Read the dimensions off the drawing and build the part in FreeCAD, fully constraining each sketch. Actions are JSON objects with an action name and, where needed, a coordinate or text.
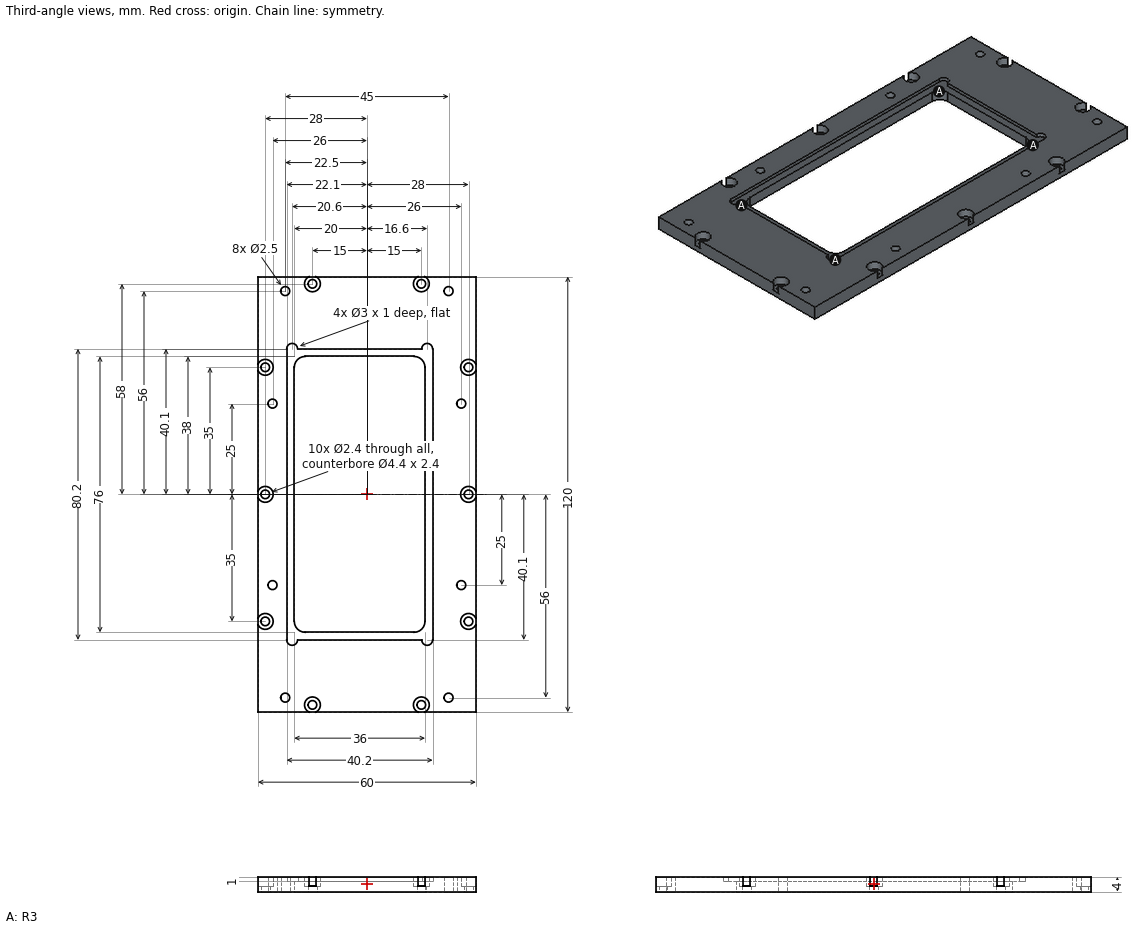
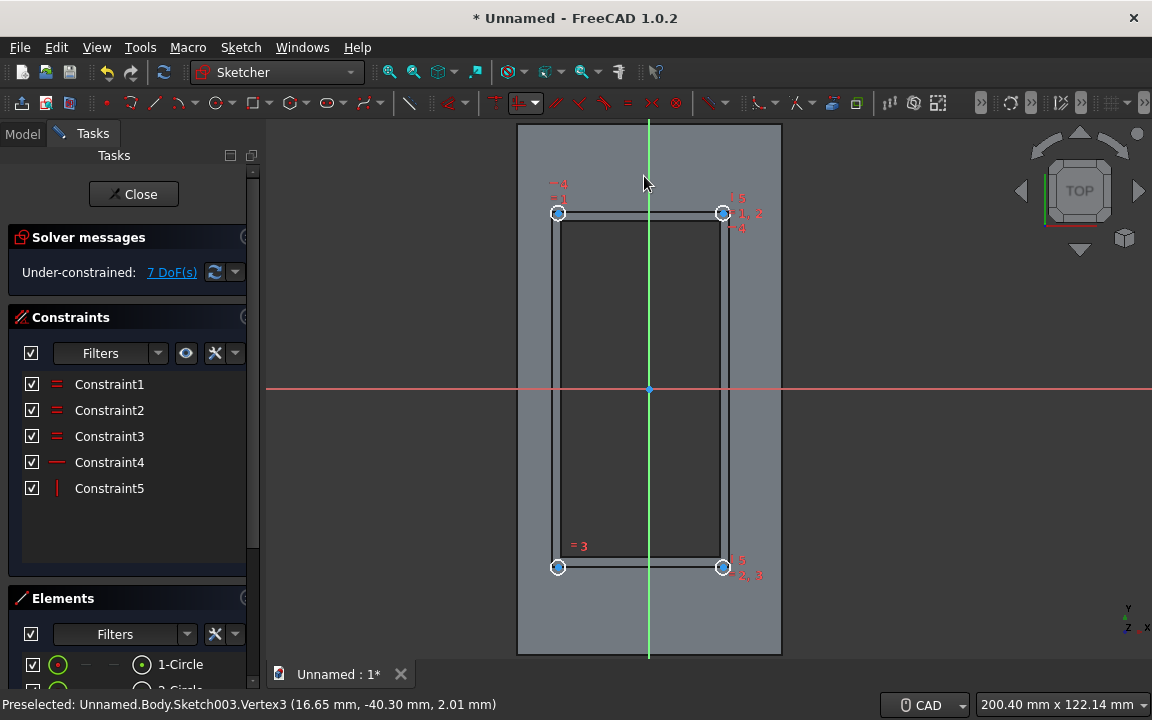
{"action": "left_click", "coordinate": [558, 213]}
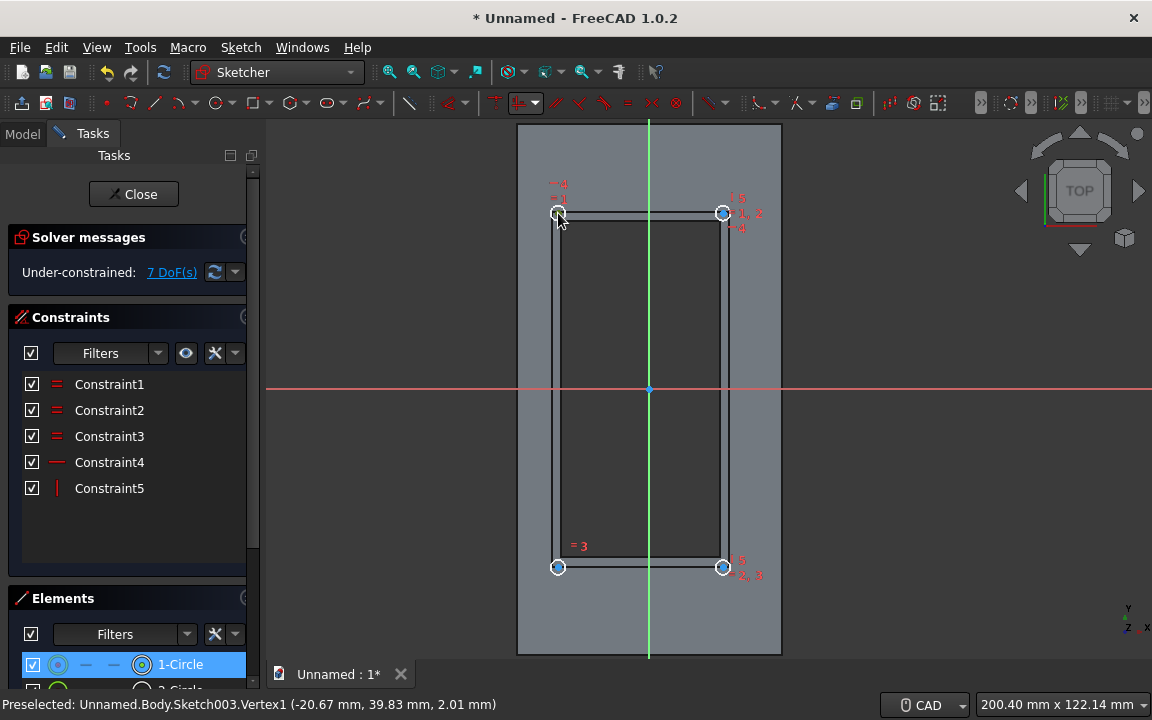
{"action": "left_click", "coordinate": [558, 567]}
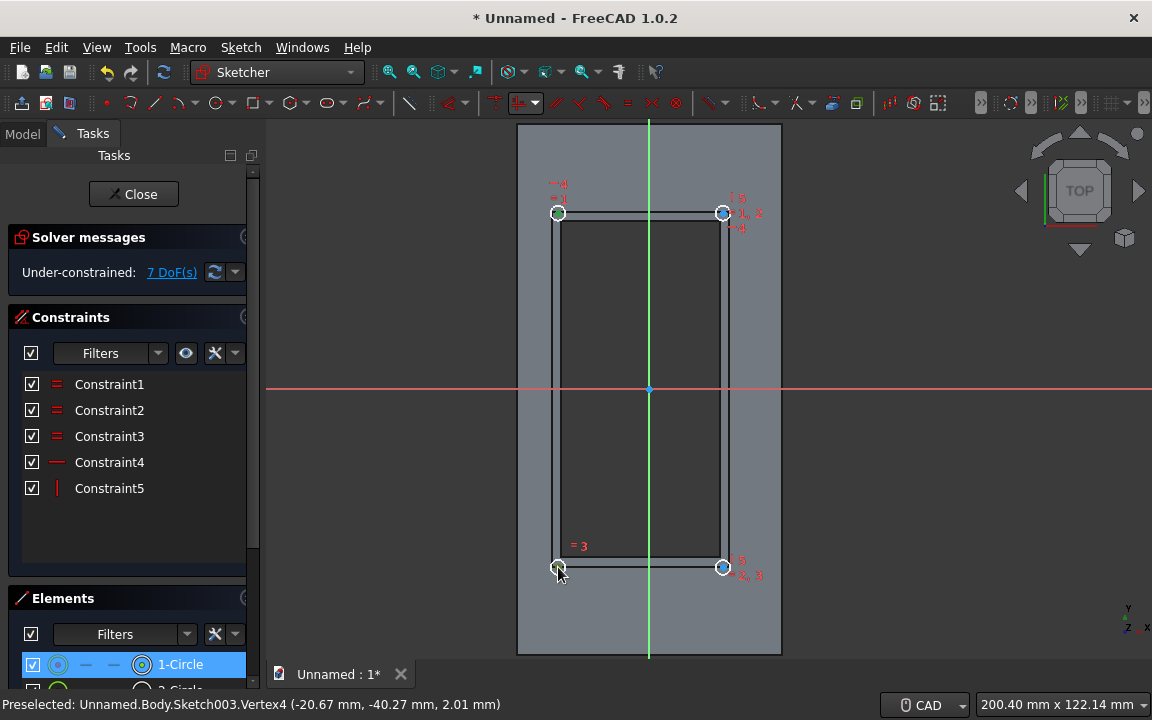
{"action": "key", "text": "v"}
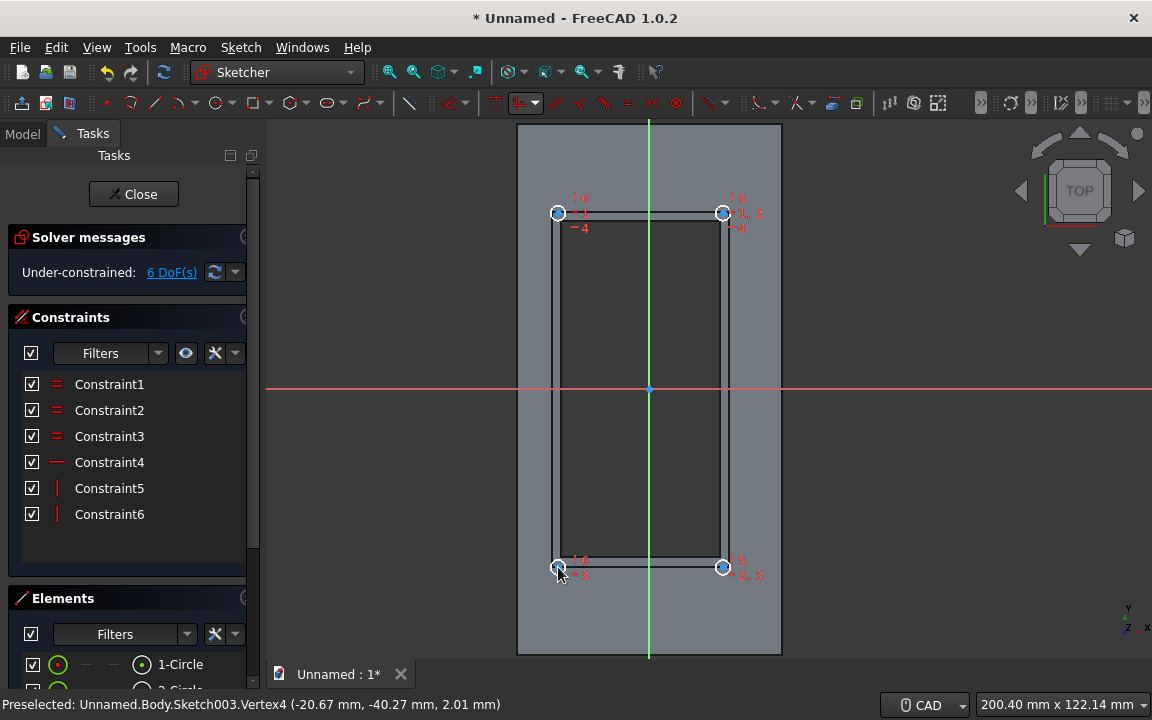
{"action": "left_click", "coordinate": [723, 567]}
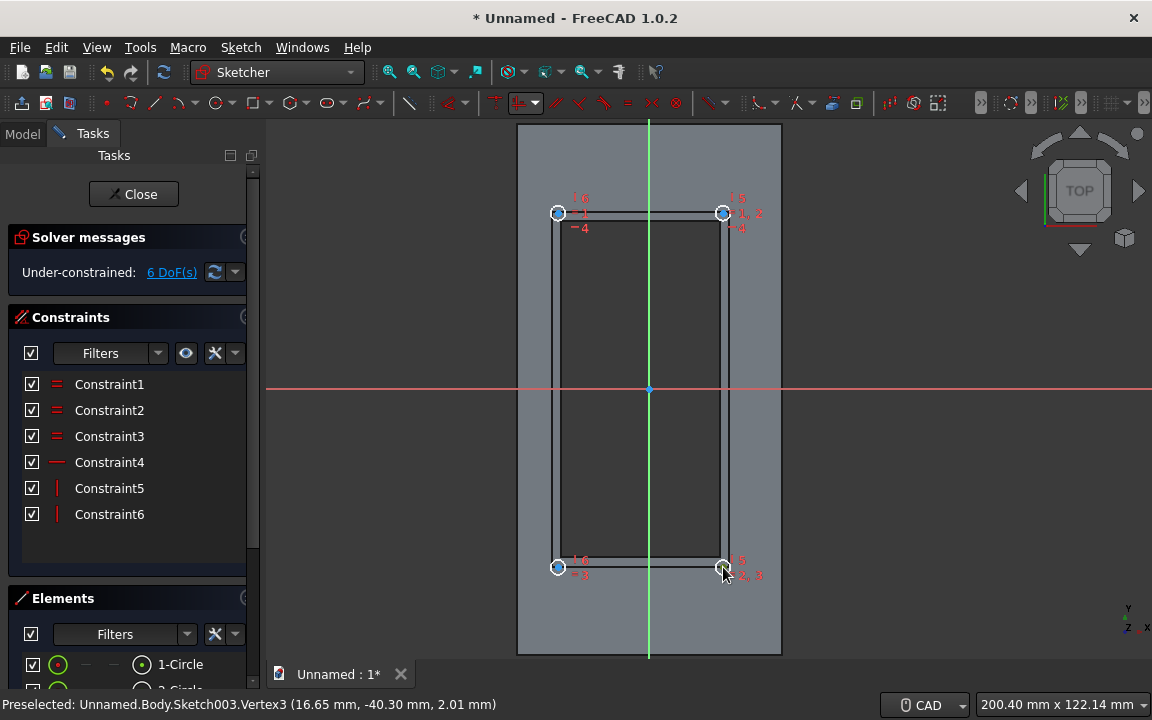
{"action": "left_click", "coordinate": [558, 567]}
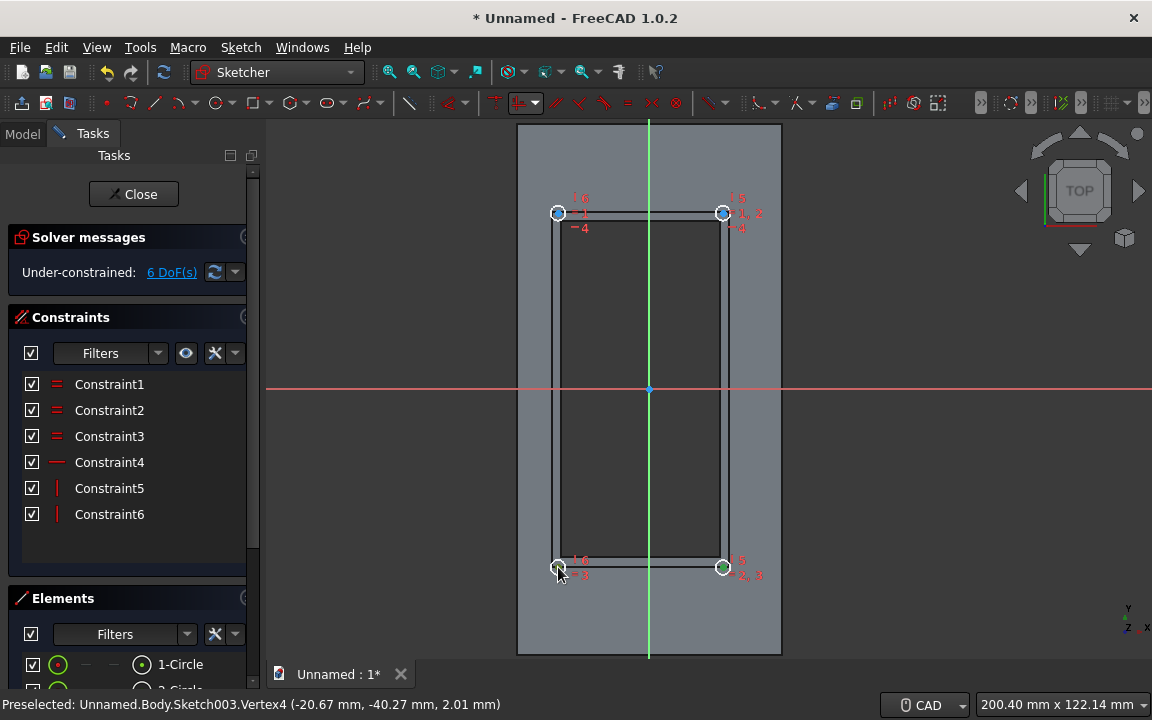
{"action": "key", "text": "h"}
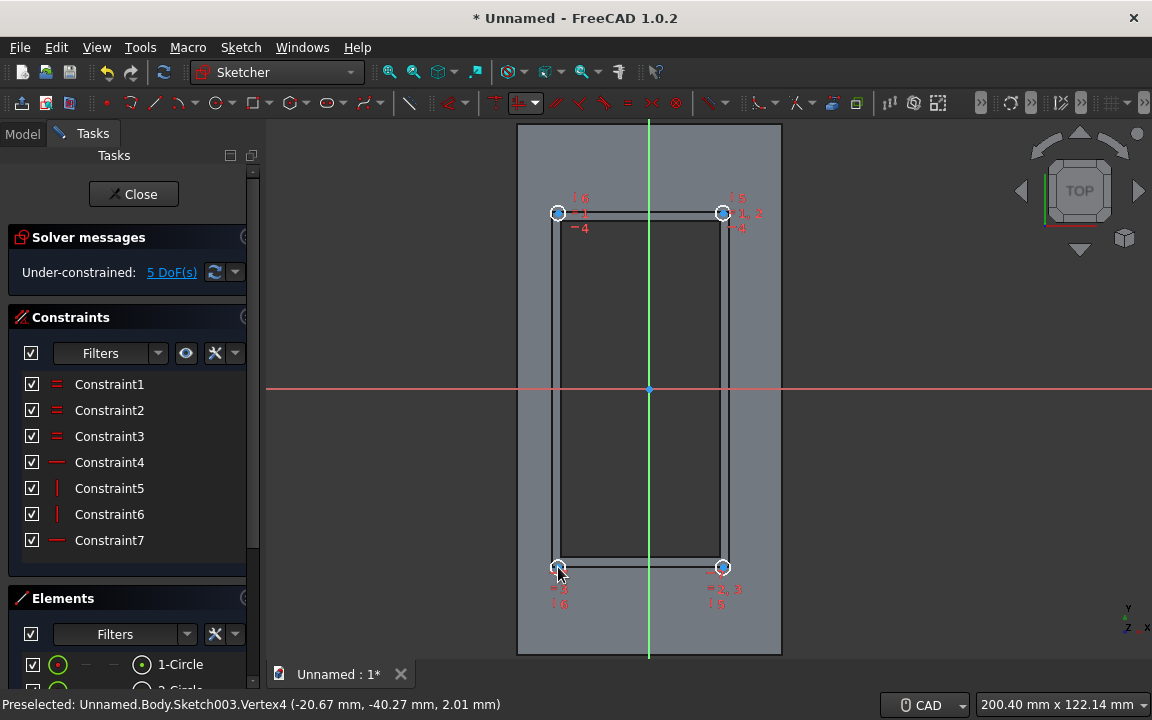
{"action": "key", "text": "d"}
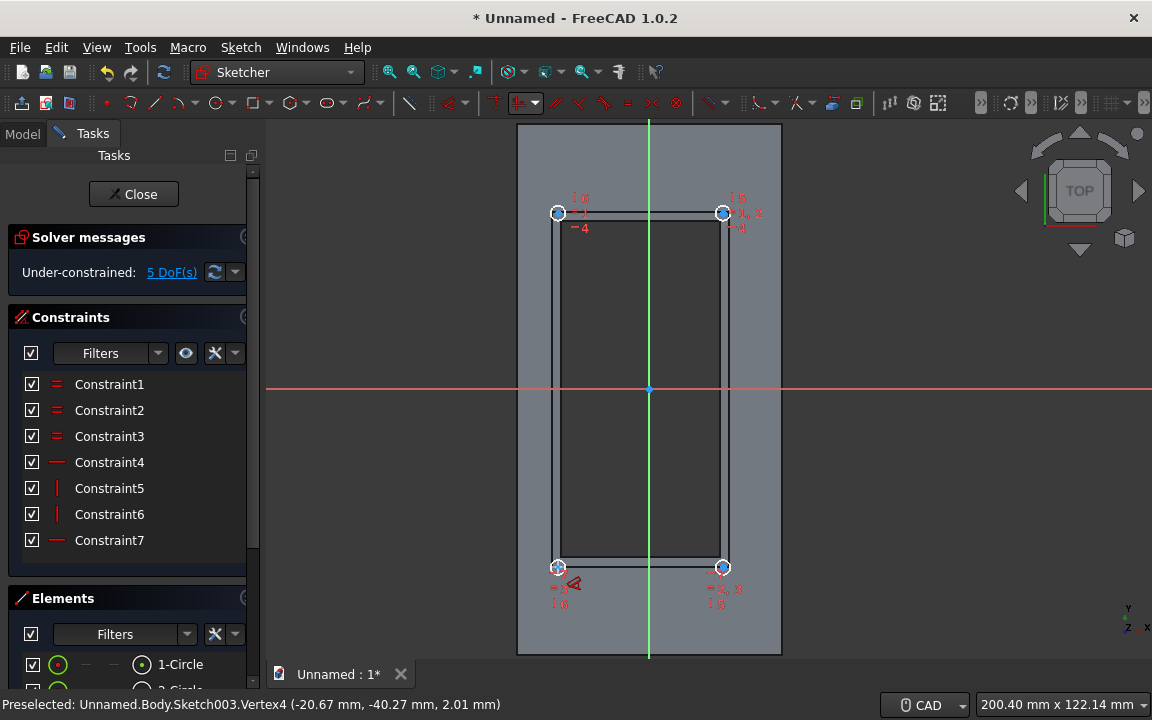
{"action": "scroll", "coordinate": [563, 218], "scroll_direction": "up", "scroll_amount": 6}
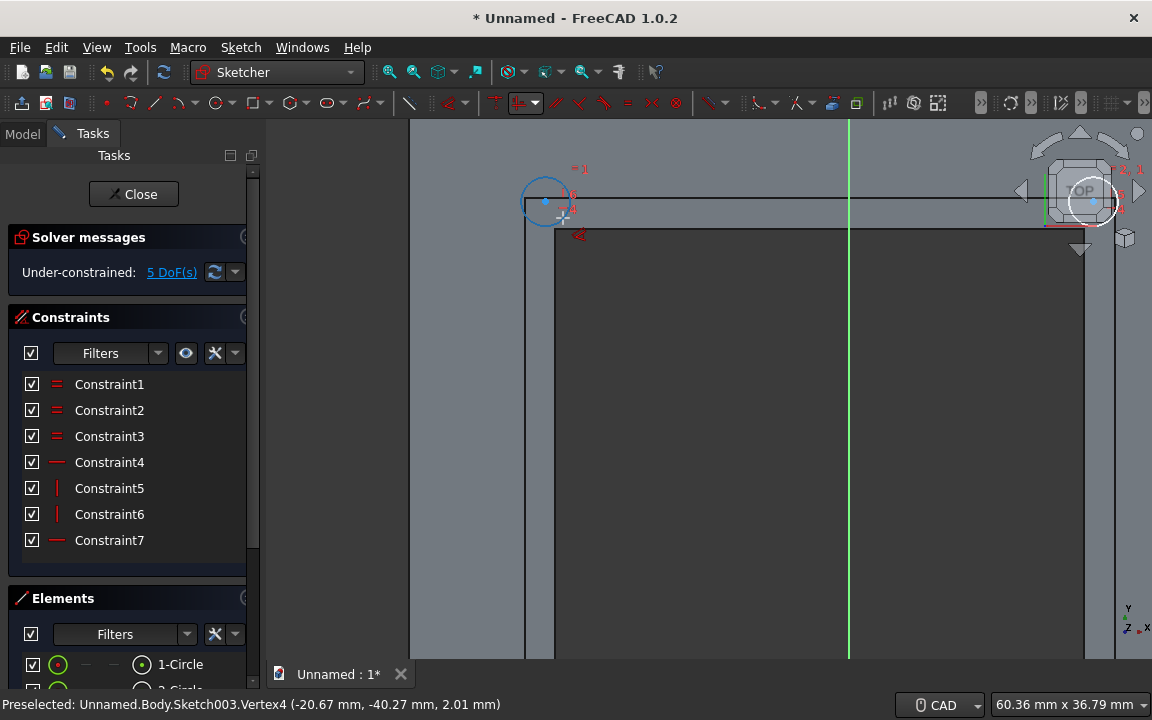
{"action": "left_click", "coordinate": [563, 219]}
{"action": "left_click", "coordinate": [586, 242]}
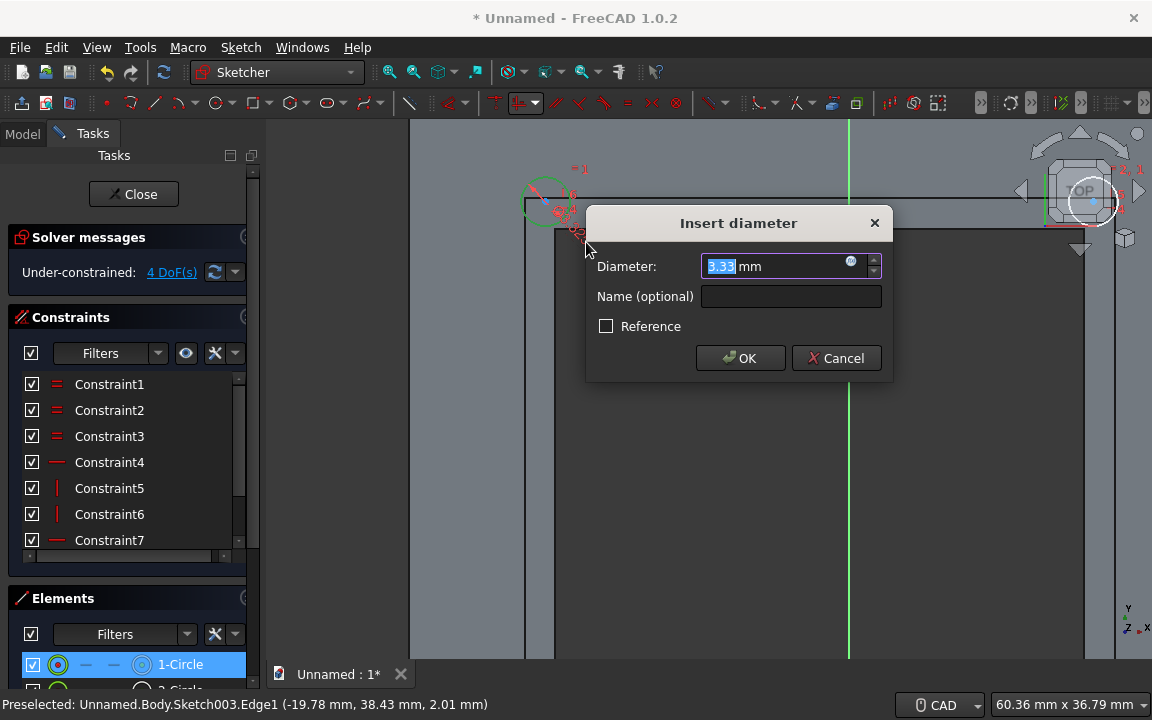
{"action": "type", "text": "3"}
{"action": "key", "text": "Return"}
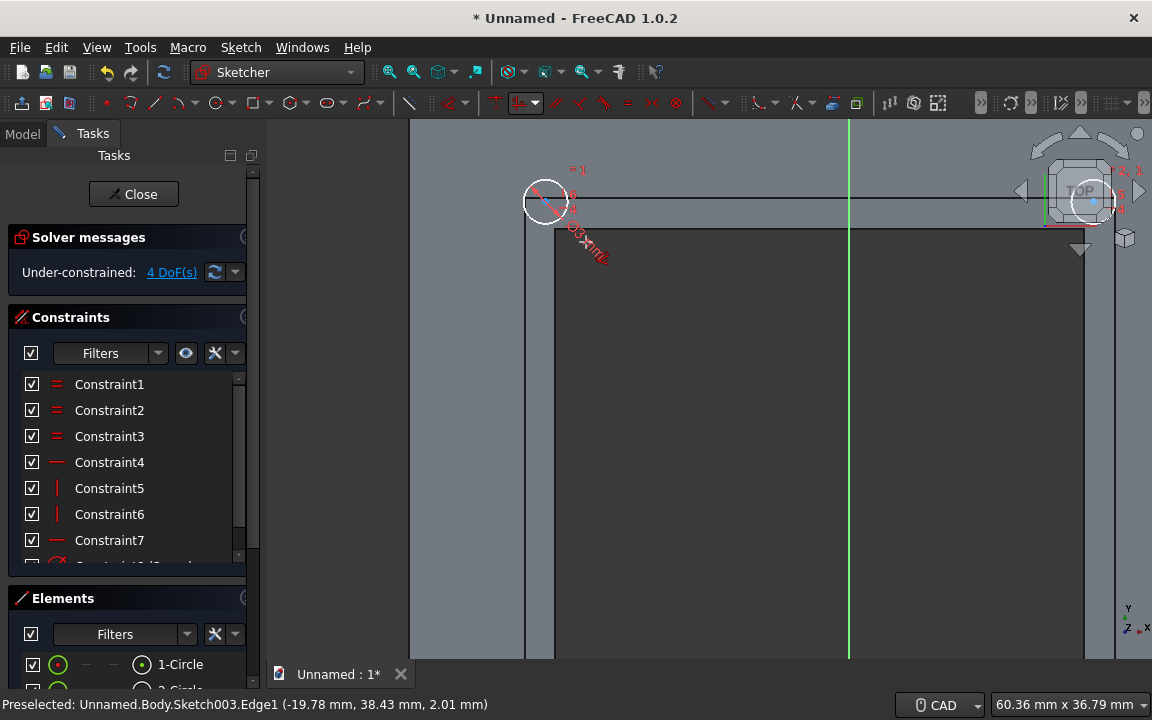
{"action": "left_click", "coordinate": [546, 202]}
{"action": "left_click", "coordinate": [697, 168]}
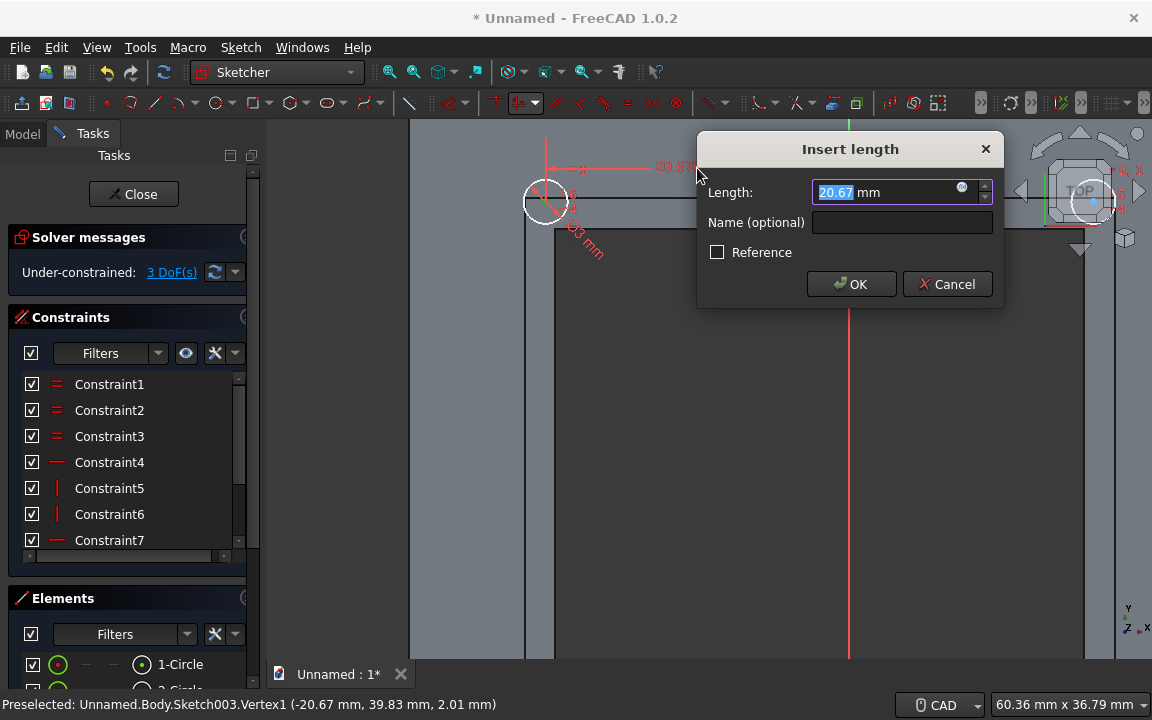
{"action": "type", "text": "20.6"}
{"action": "key", "text": "Return"}